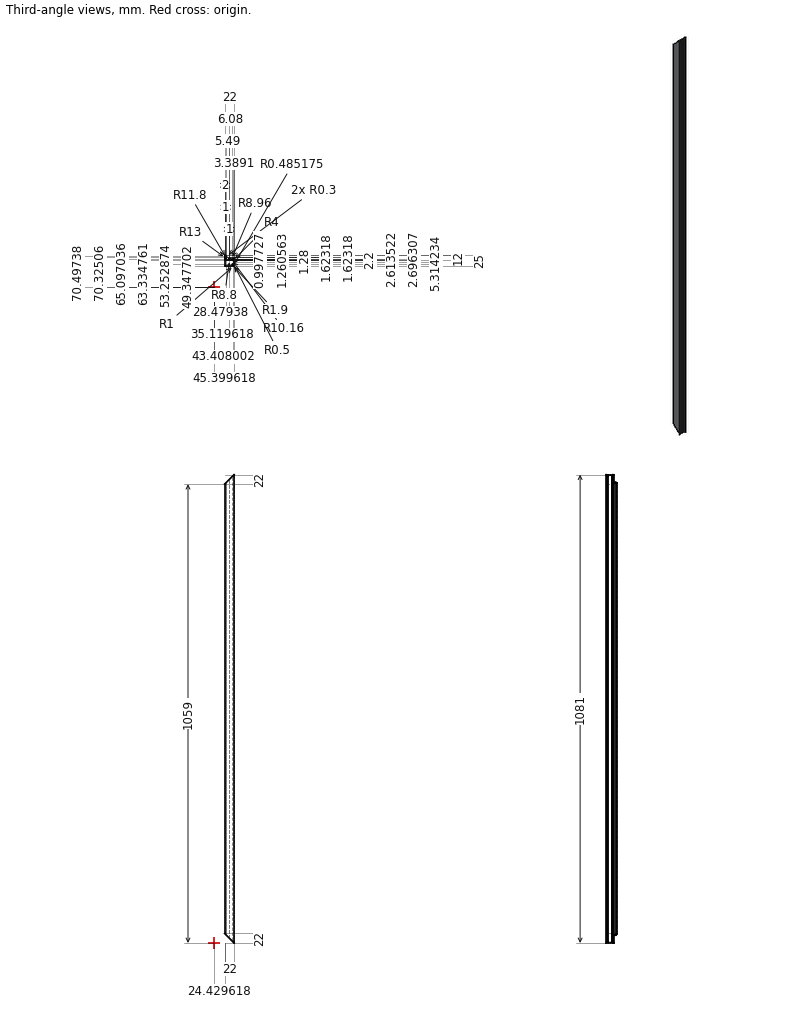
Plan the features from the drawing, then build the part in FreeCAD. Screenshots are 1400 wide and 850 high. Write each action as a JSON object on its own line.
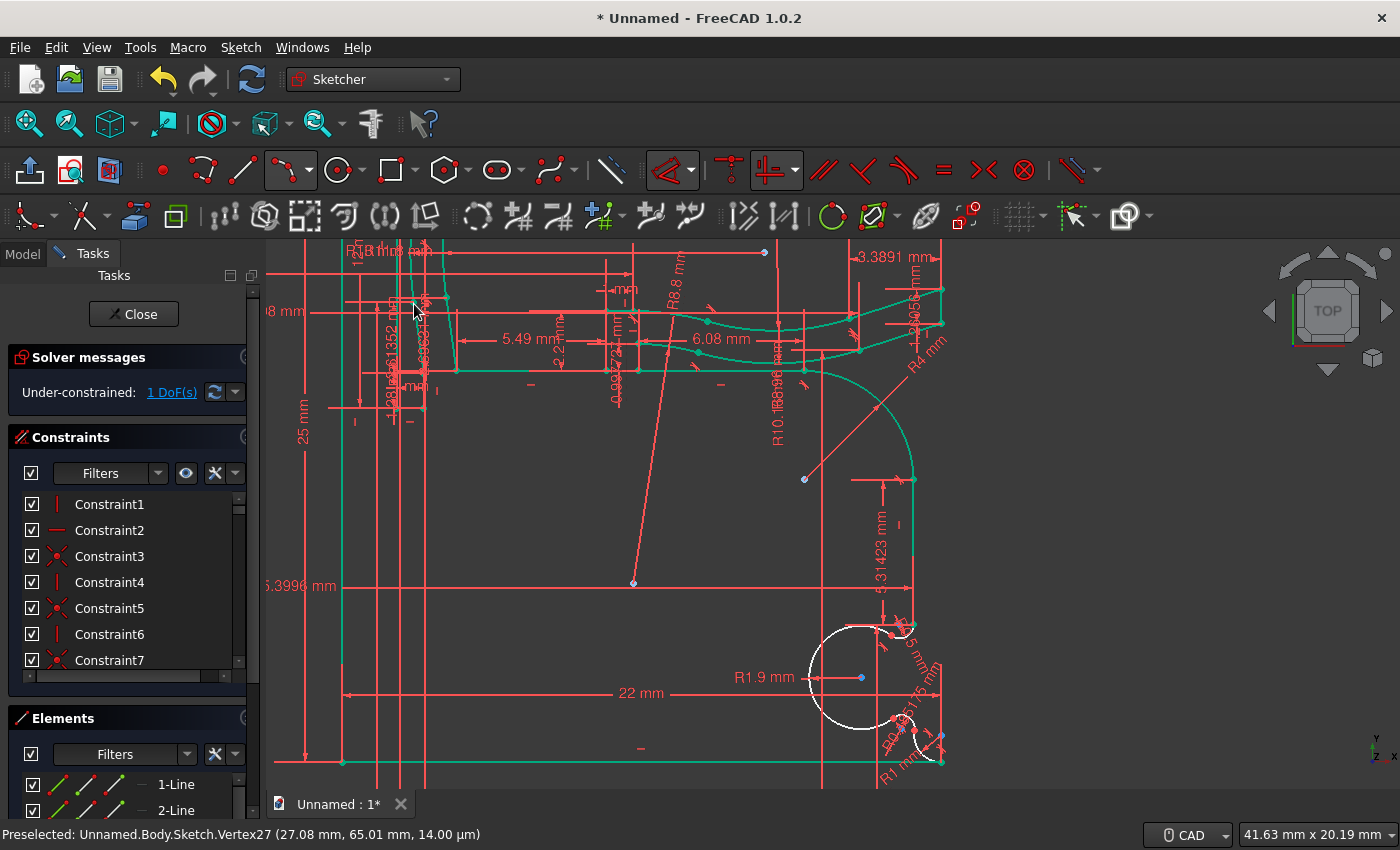
{"action": "left_click", "coordinate": [915, 731]}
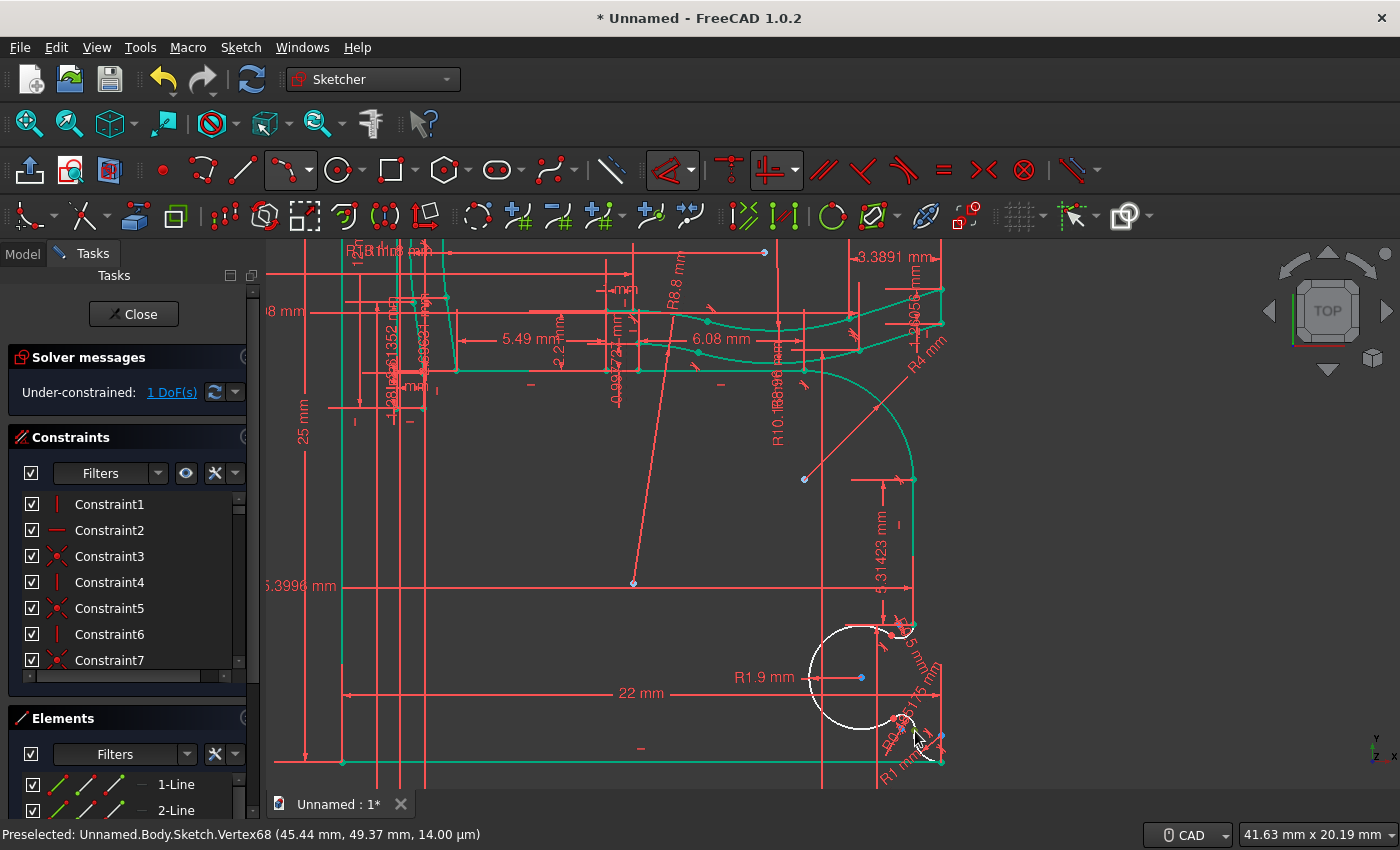
{"action": "left_click", "coordinate": [694, 170]}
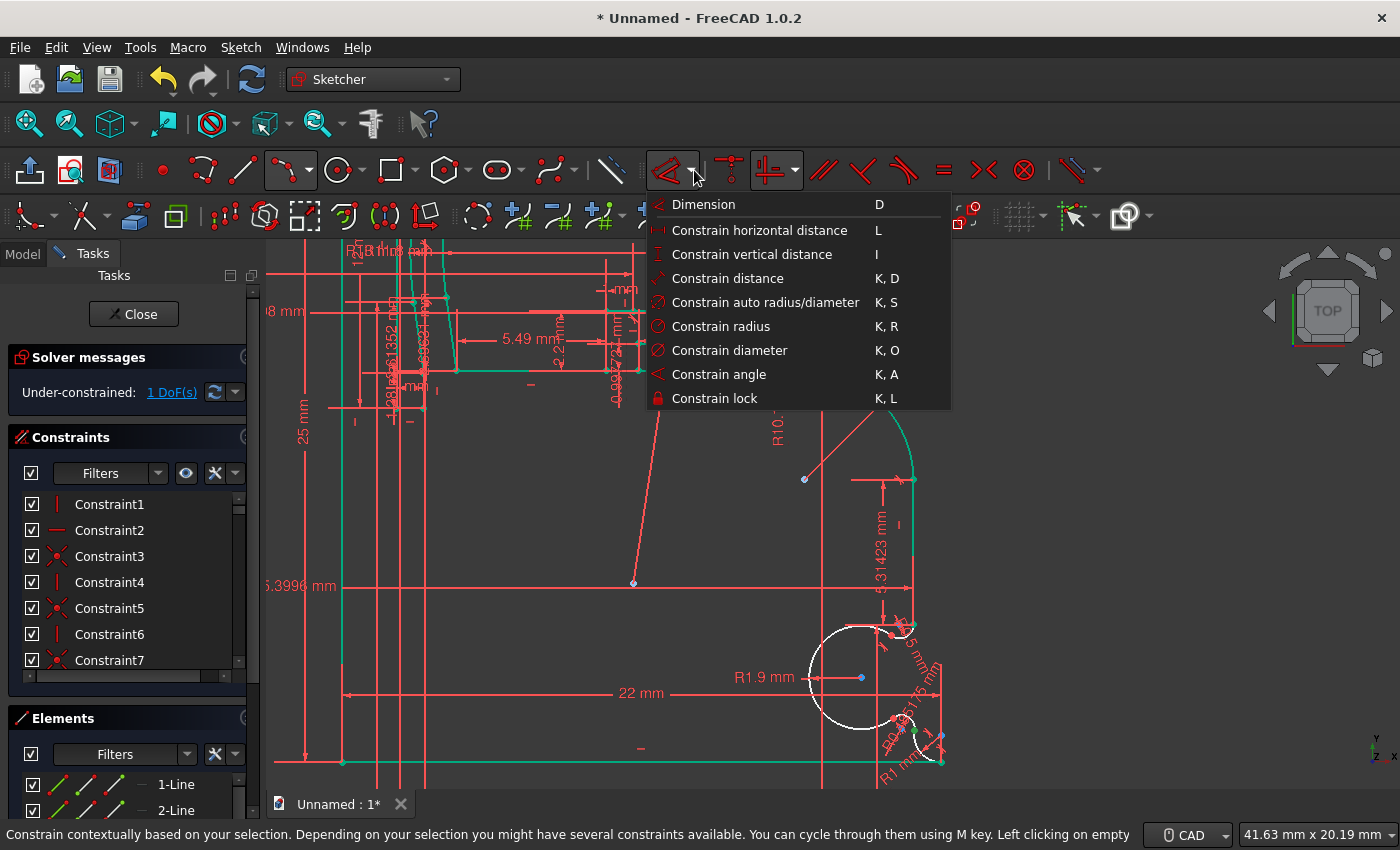
{"action": "left_click", "coordinate": [799, 254]}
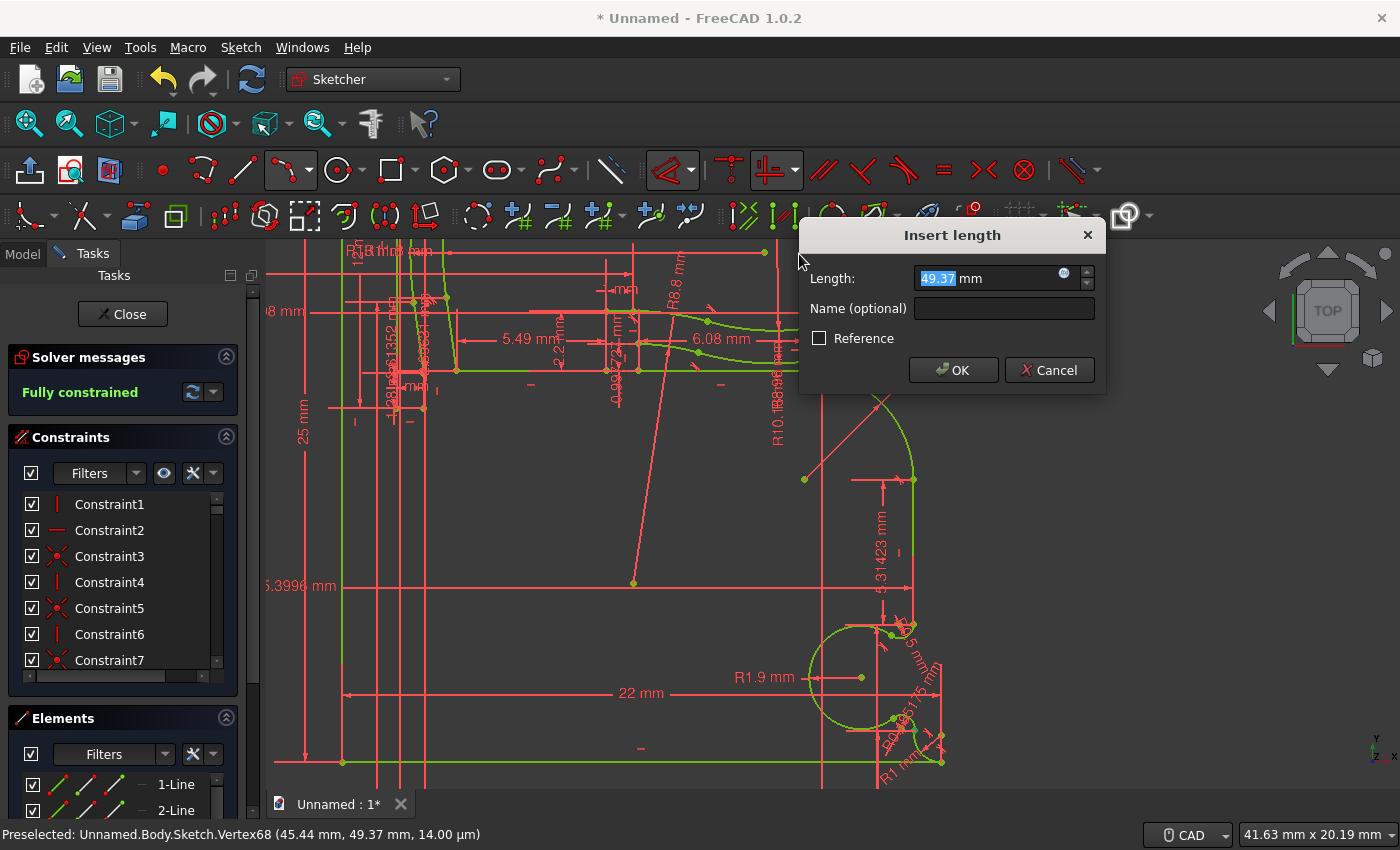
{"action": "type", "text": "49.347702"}
{"action": "key", "text": "Return"}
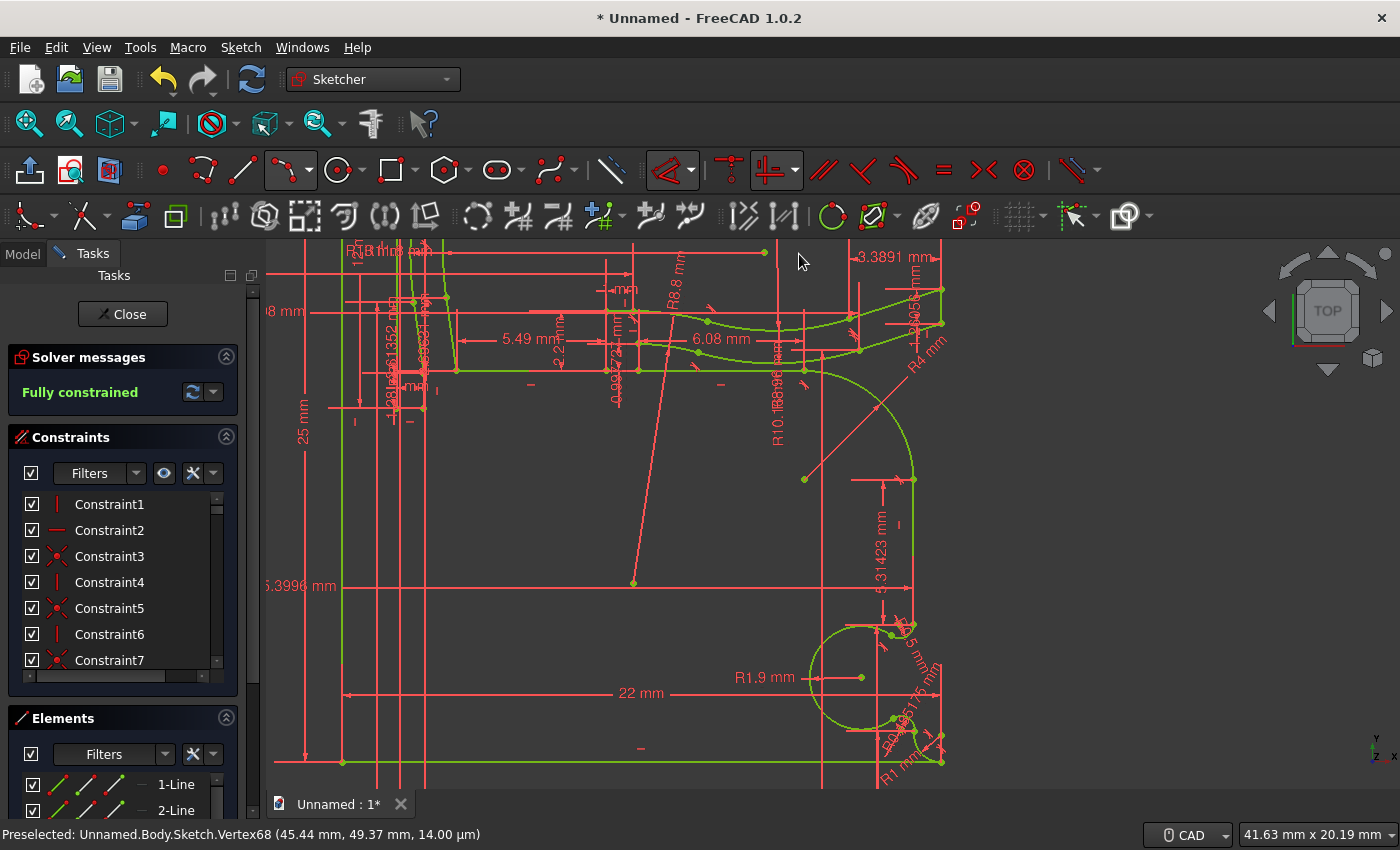
{"action": "left_click", "coordinate": [123, 314]}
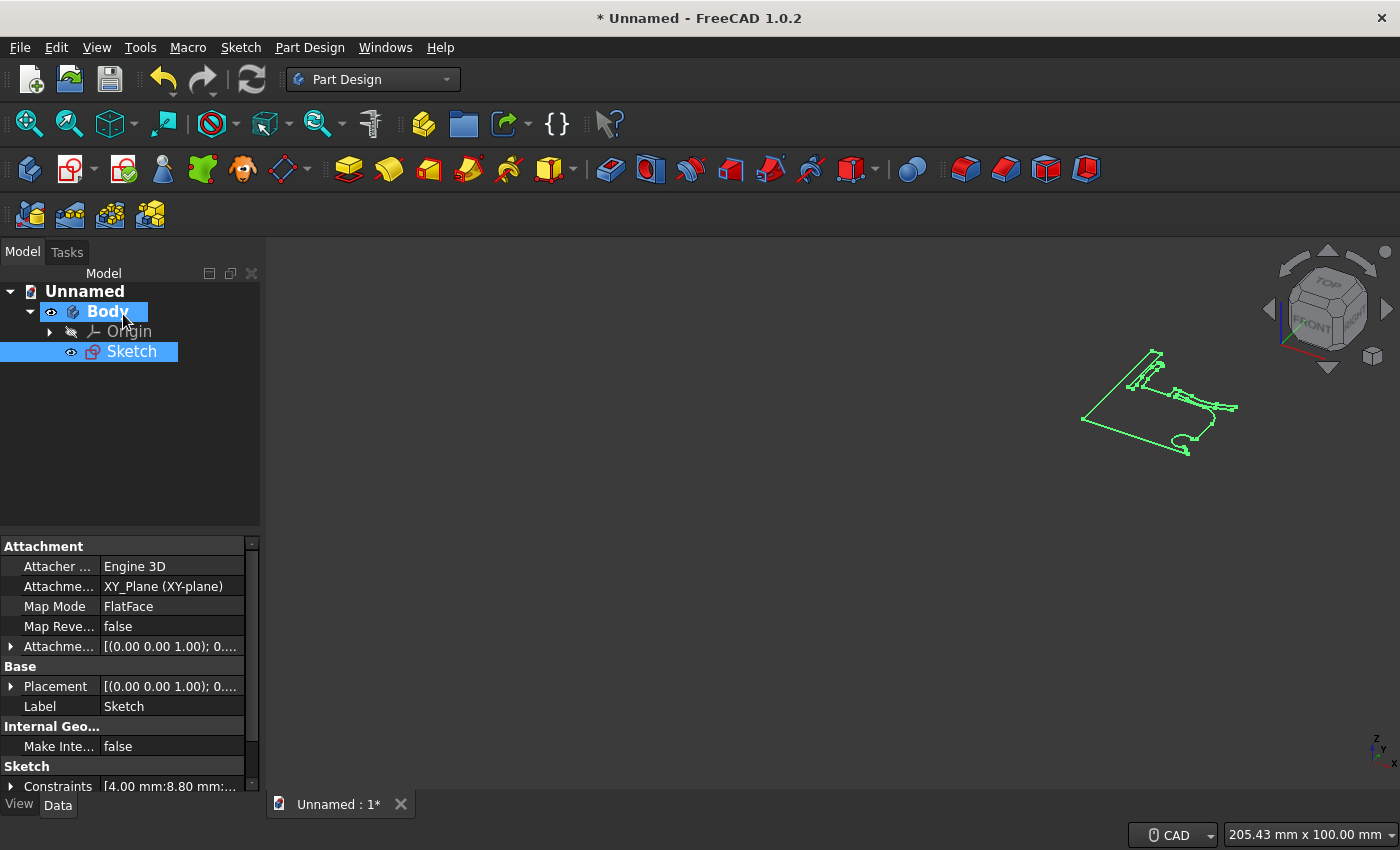
{"action": "left_click", "coordinate": [350, 170]}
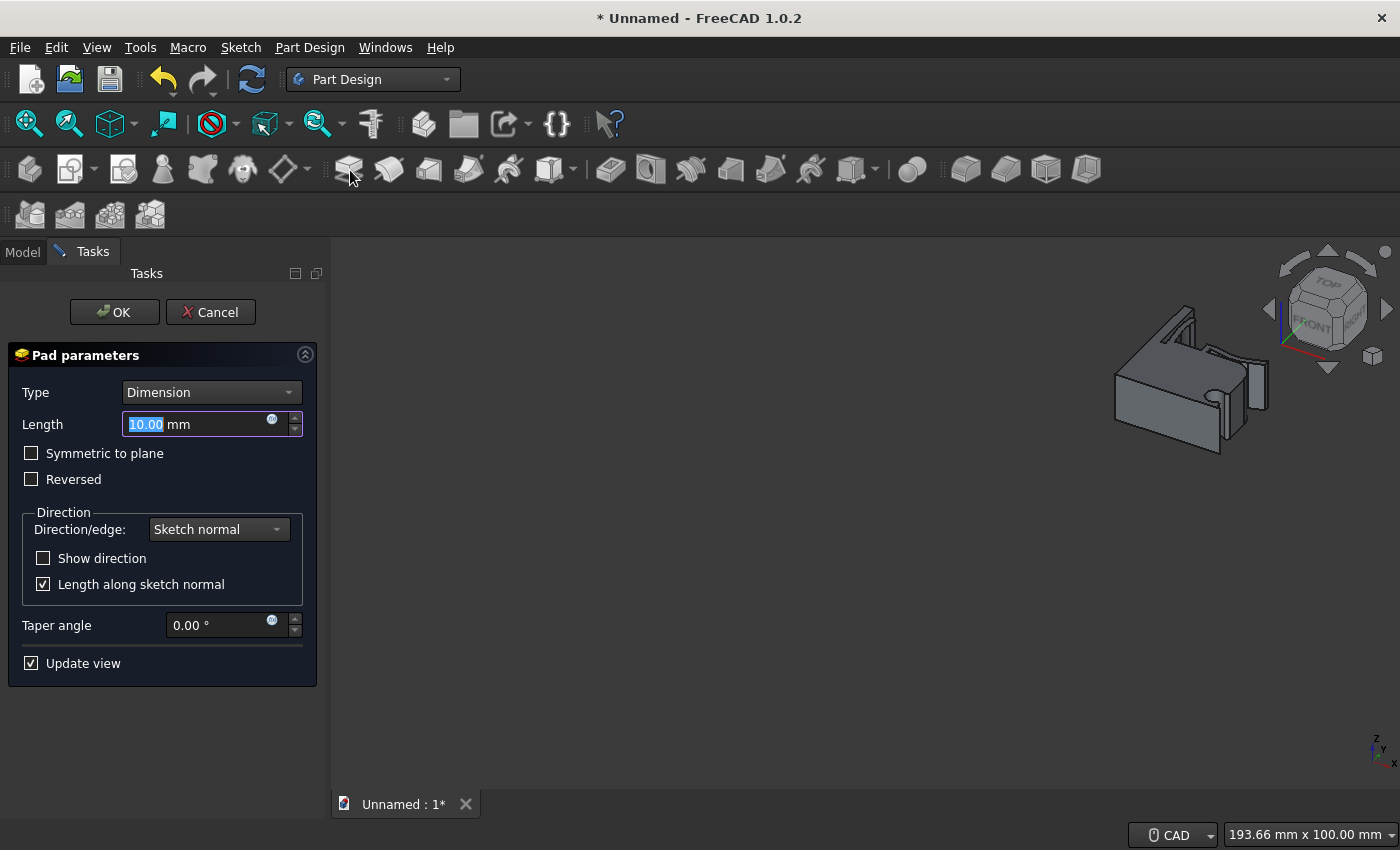
{"action": "type", "text": "1081"}
{"action": "key", "text": "Tab"}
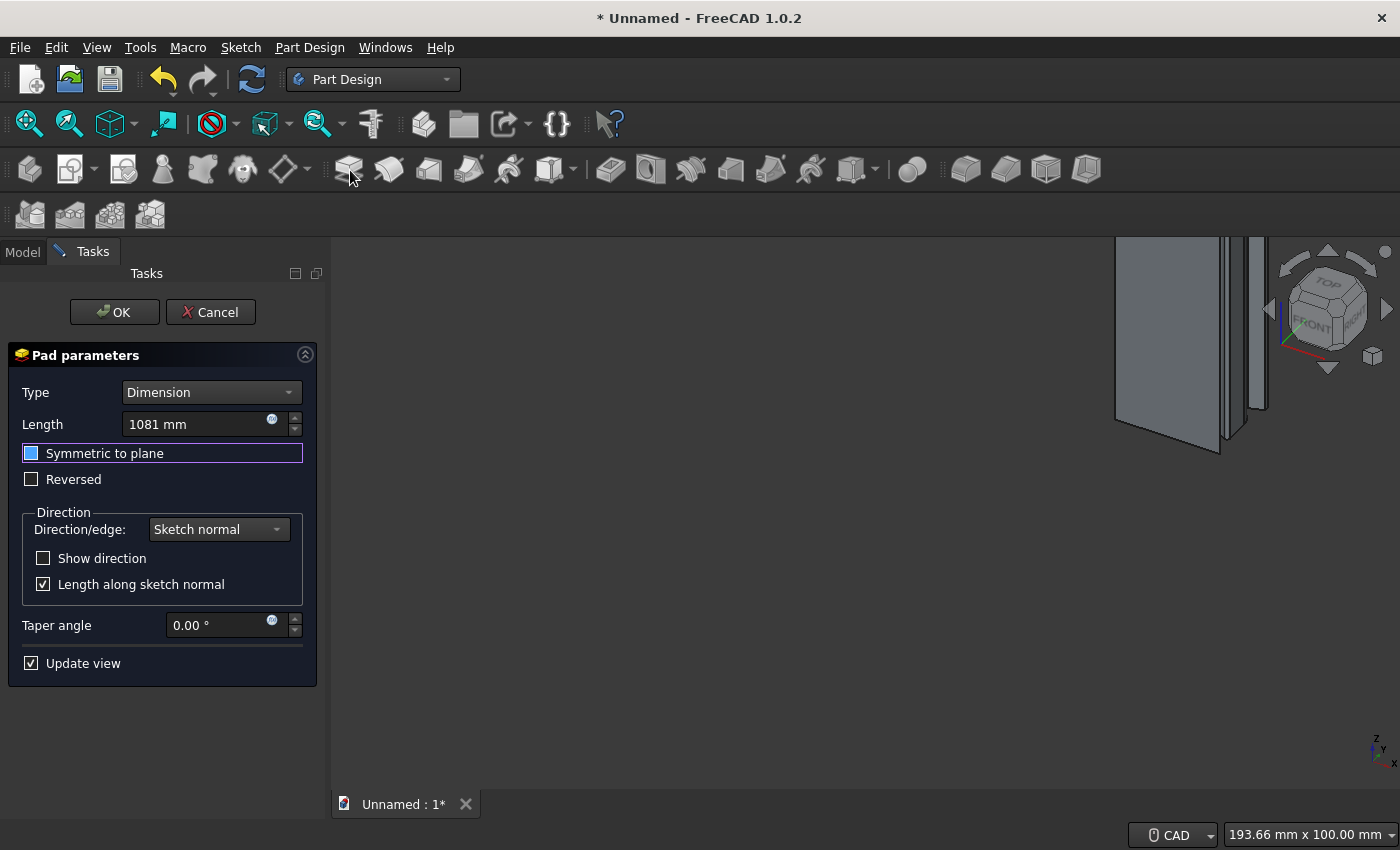
{"action": "left_click", "coordinate": [115, 312]}